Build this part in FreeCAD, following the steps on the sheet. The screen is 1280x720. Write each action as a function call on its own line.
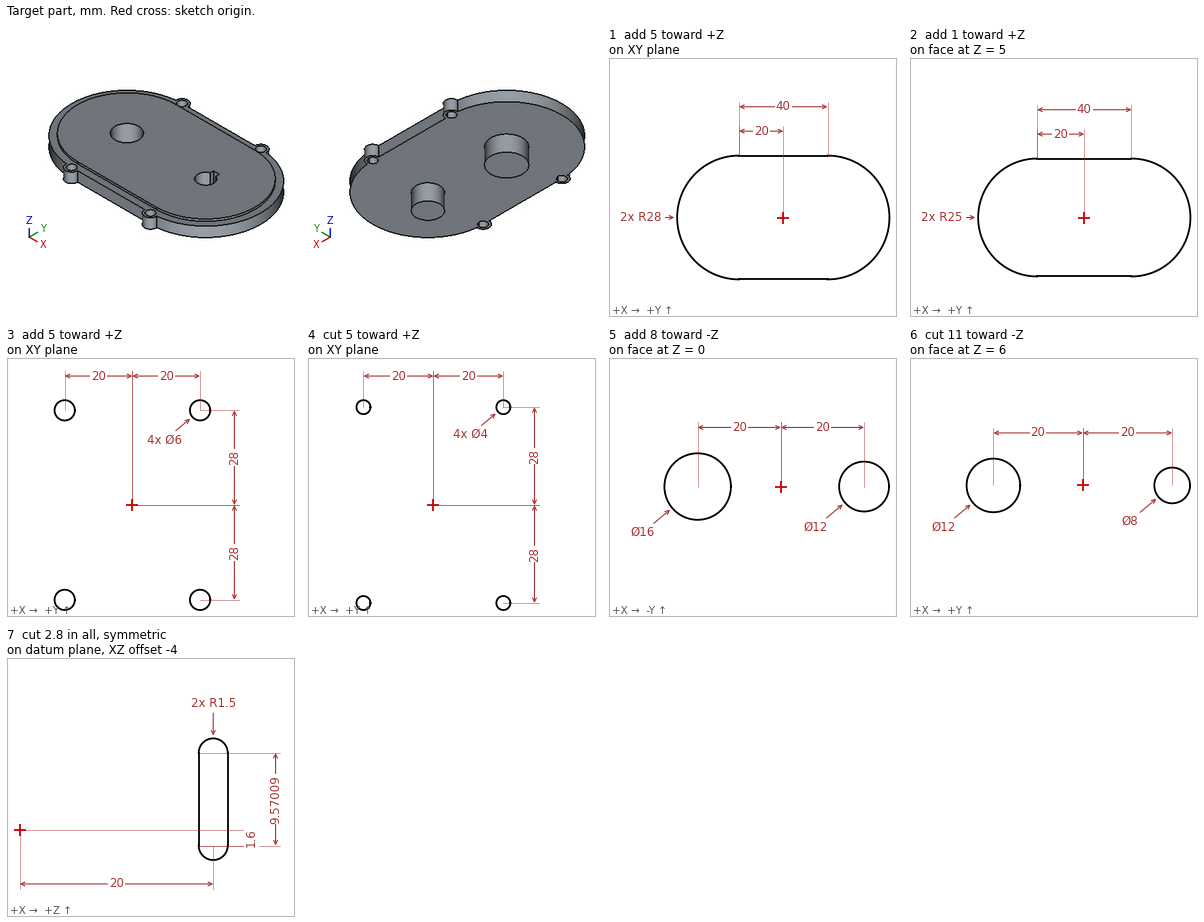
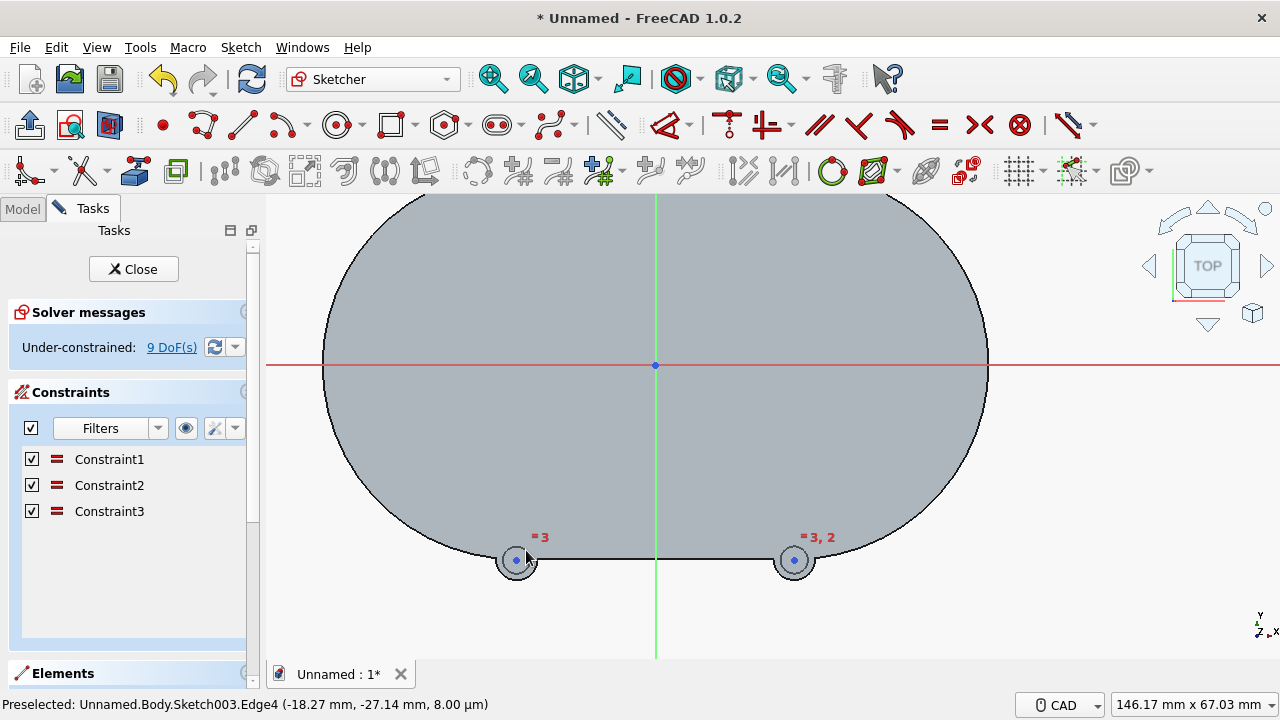
scroll(804, 551, down, 2)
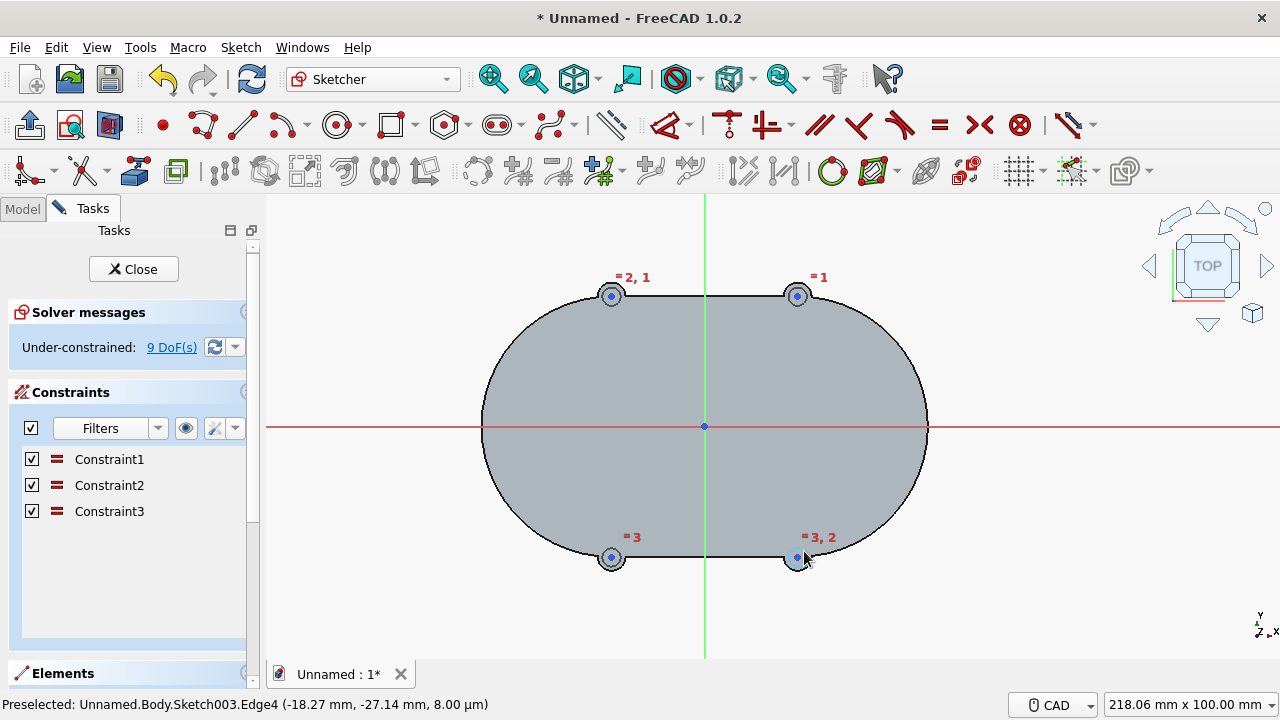
click(798, 297)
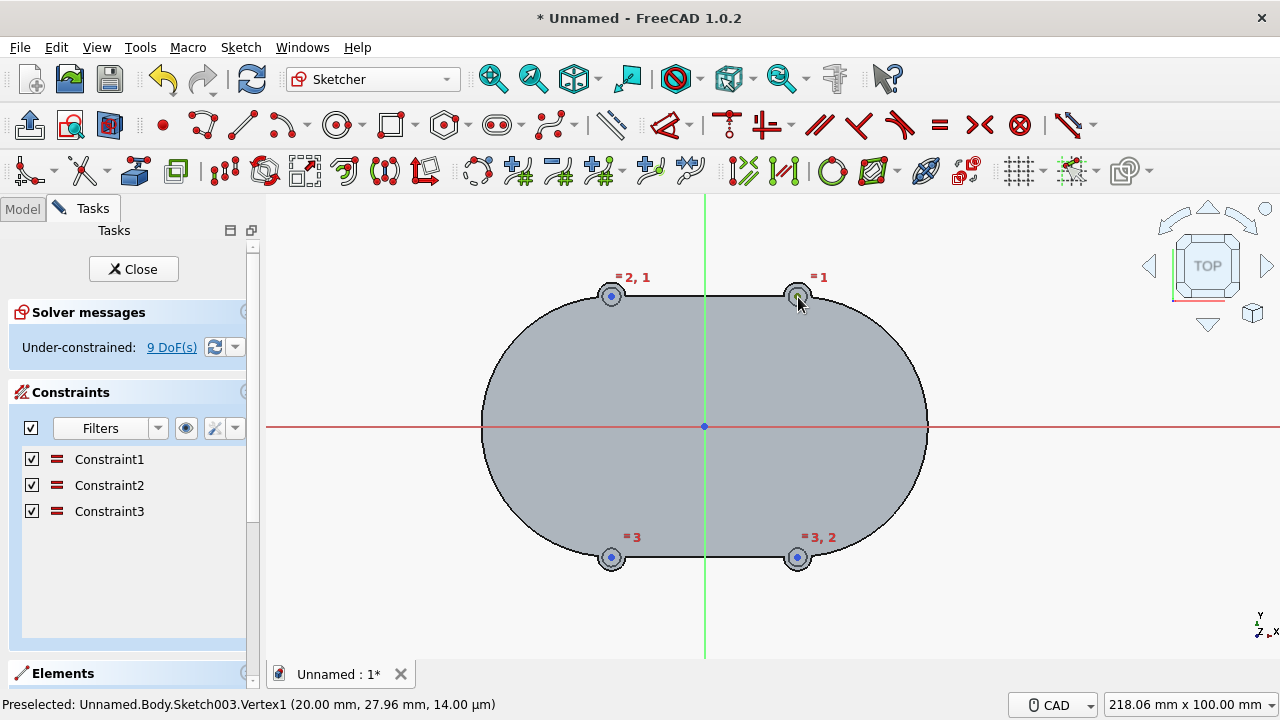
click(612, 297)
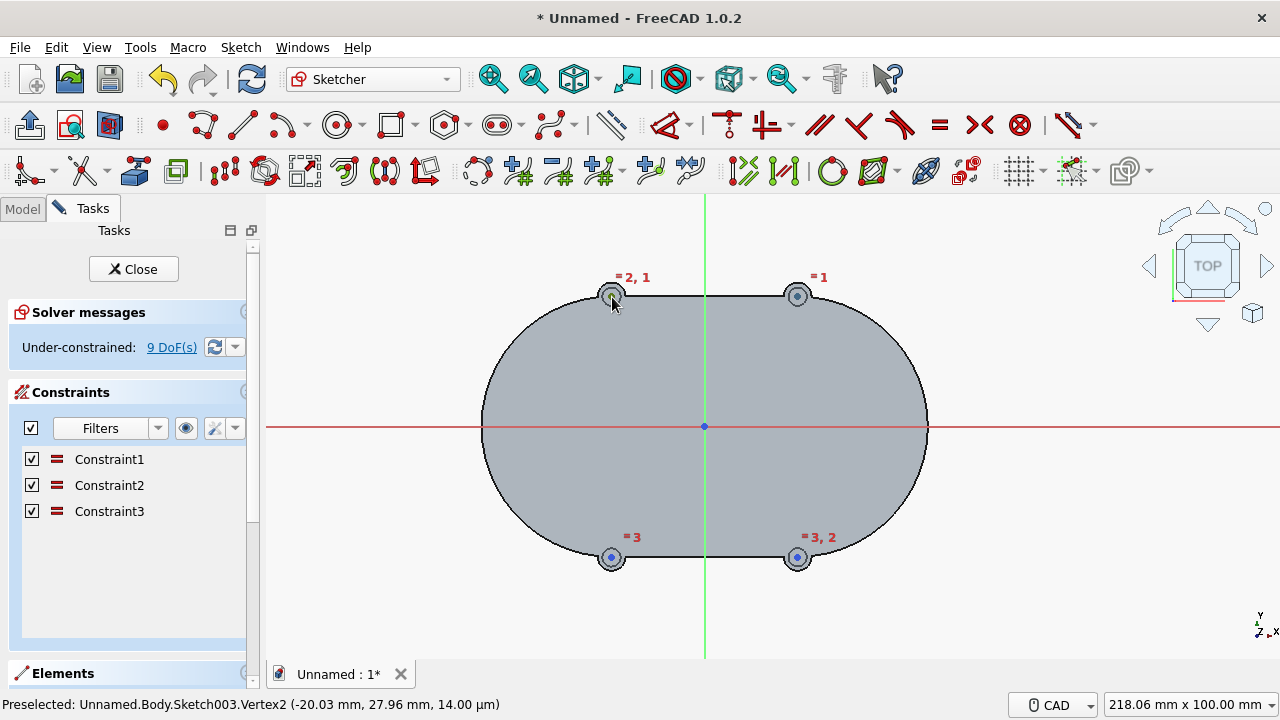
key(h)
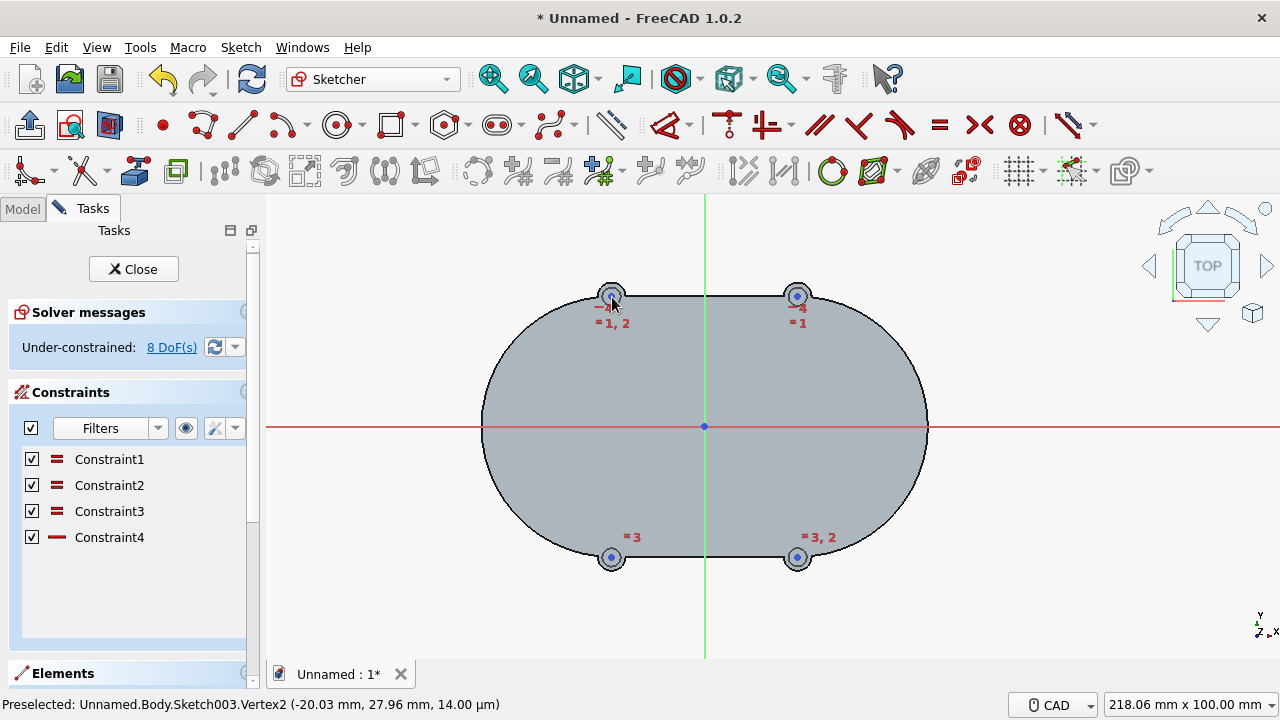
click(798, 297)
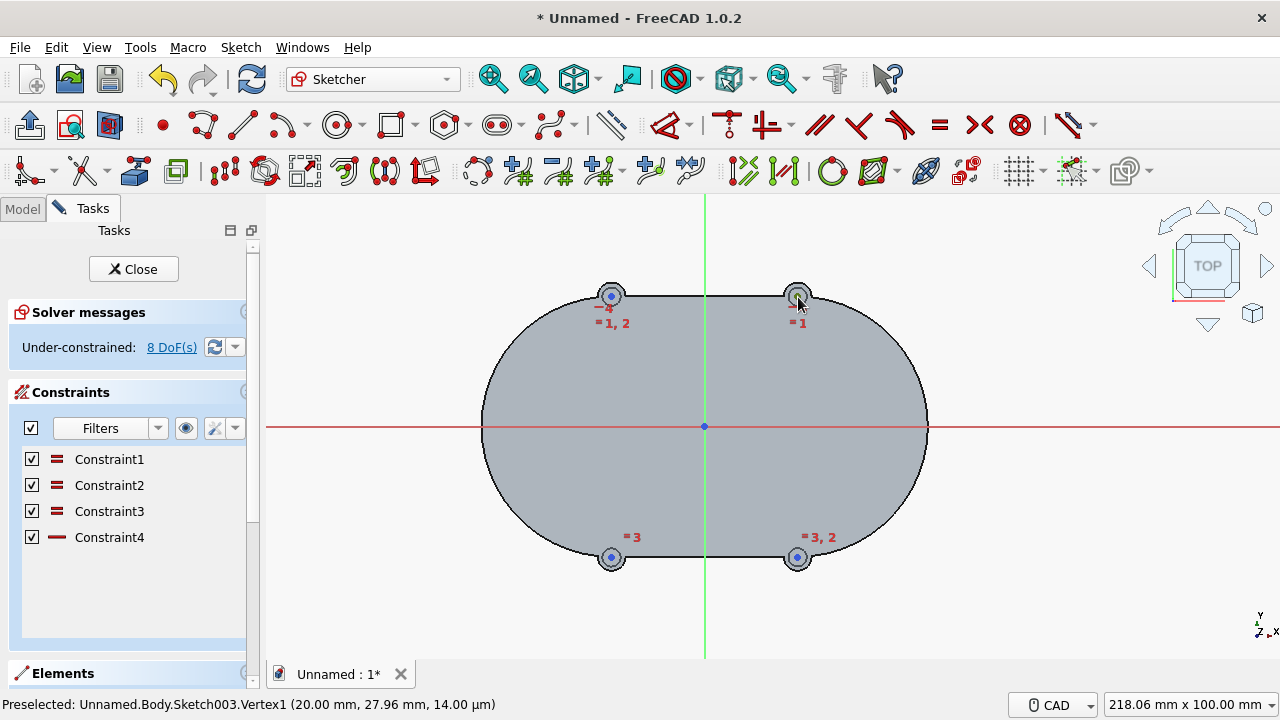
click(798, 557)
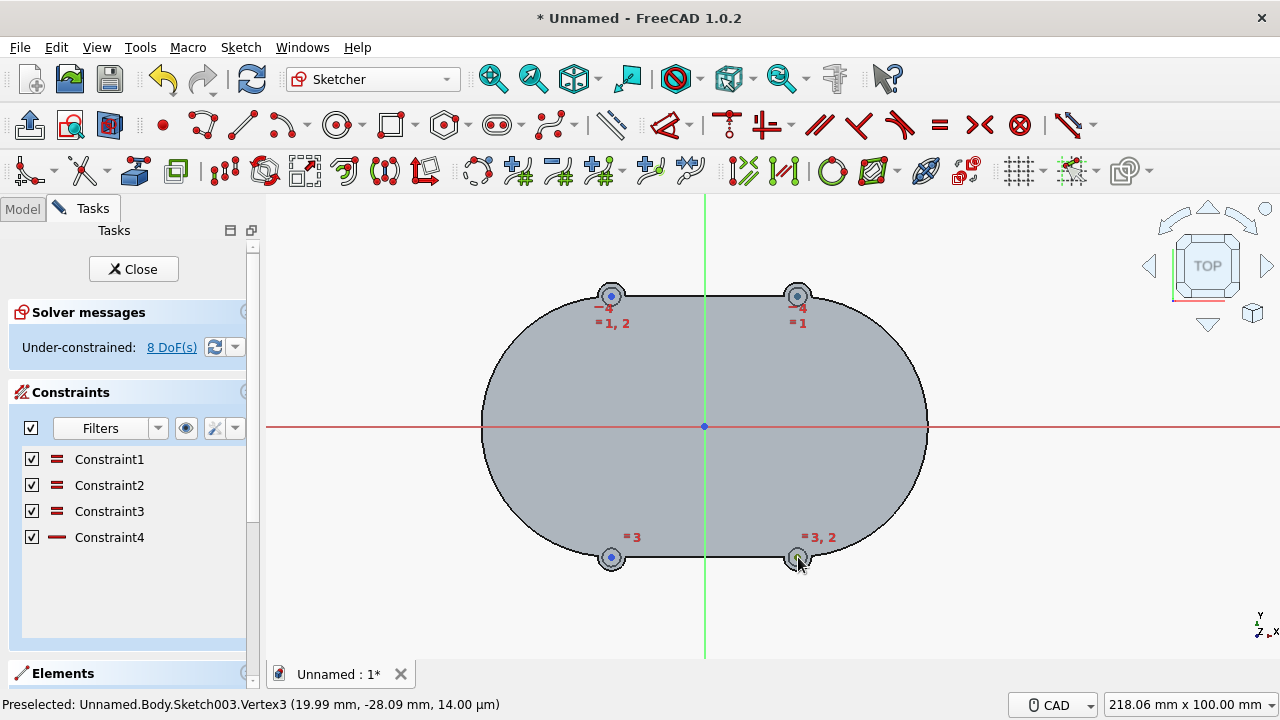
key(v)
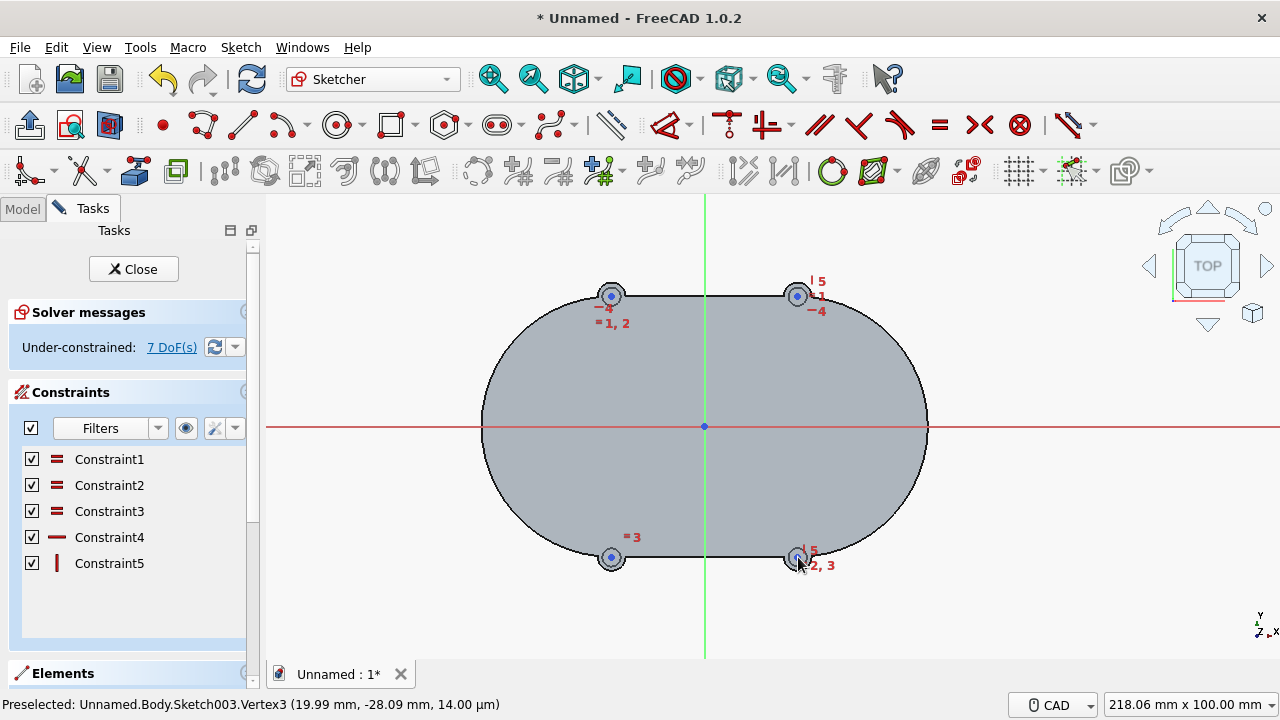
click(612, 297)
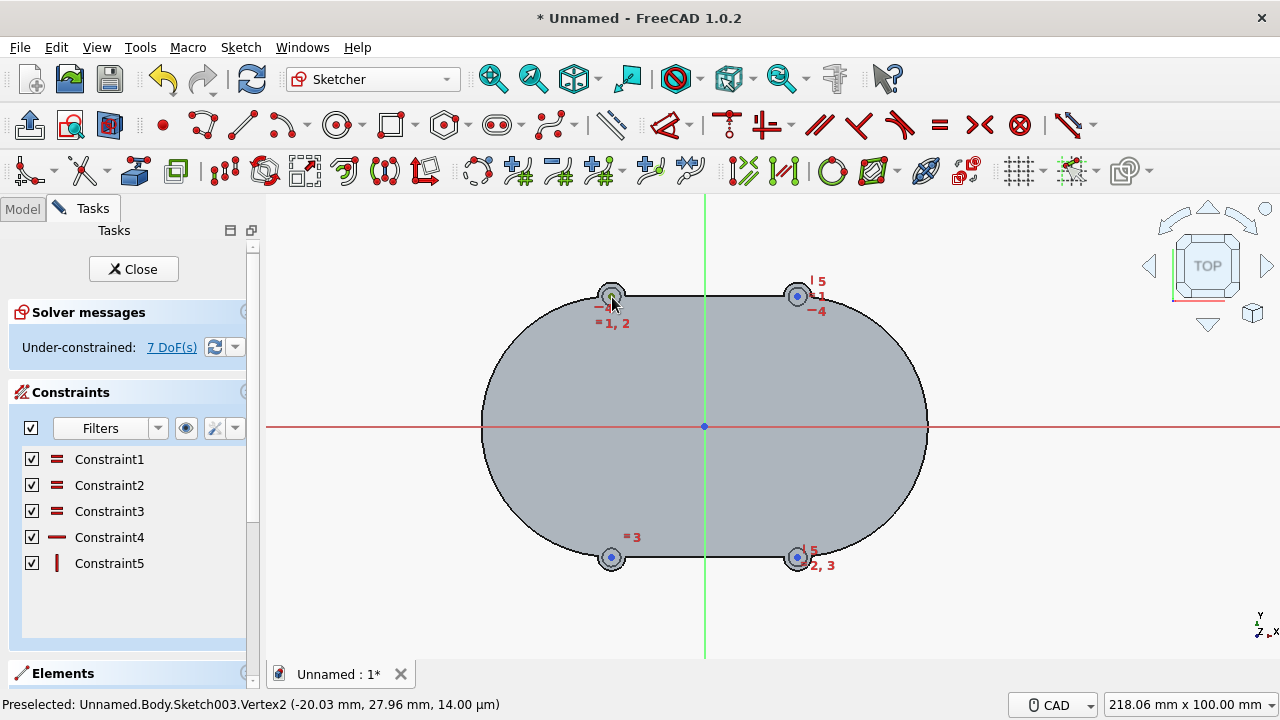
click(611, 557)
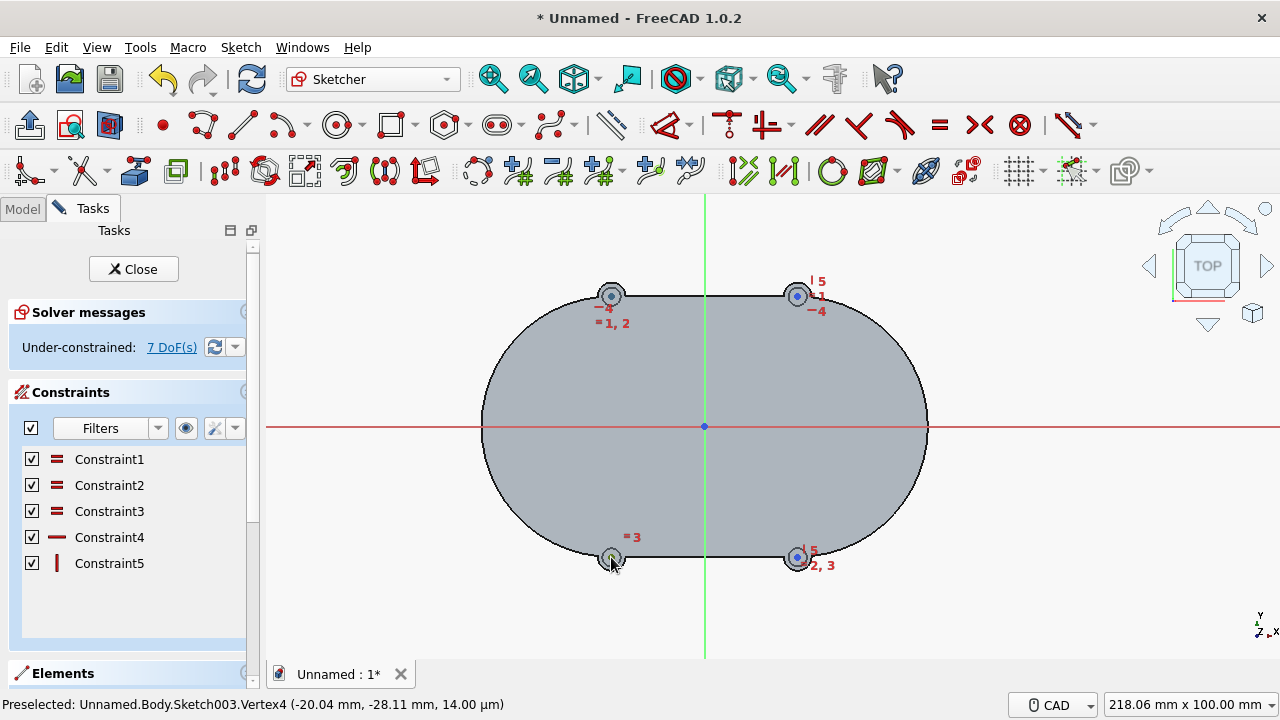
key(v)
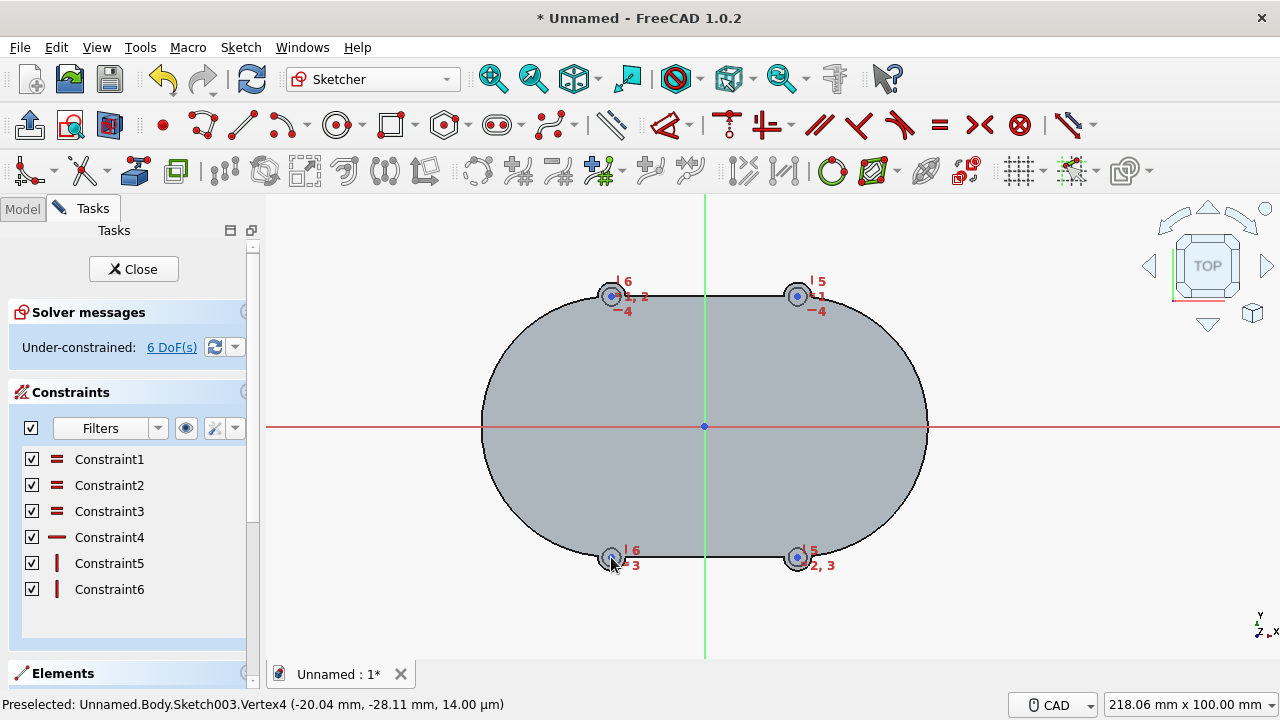
click(796, 559)